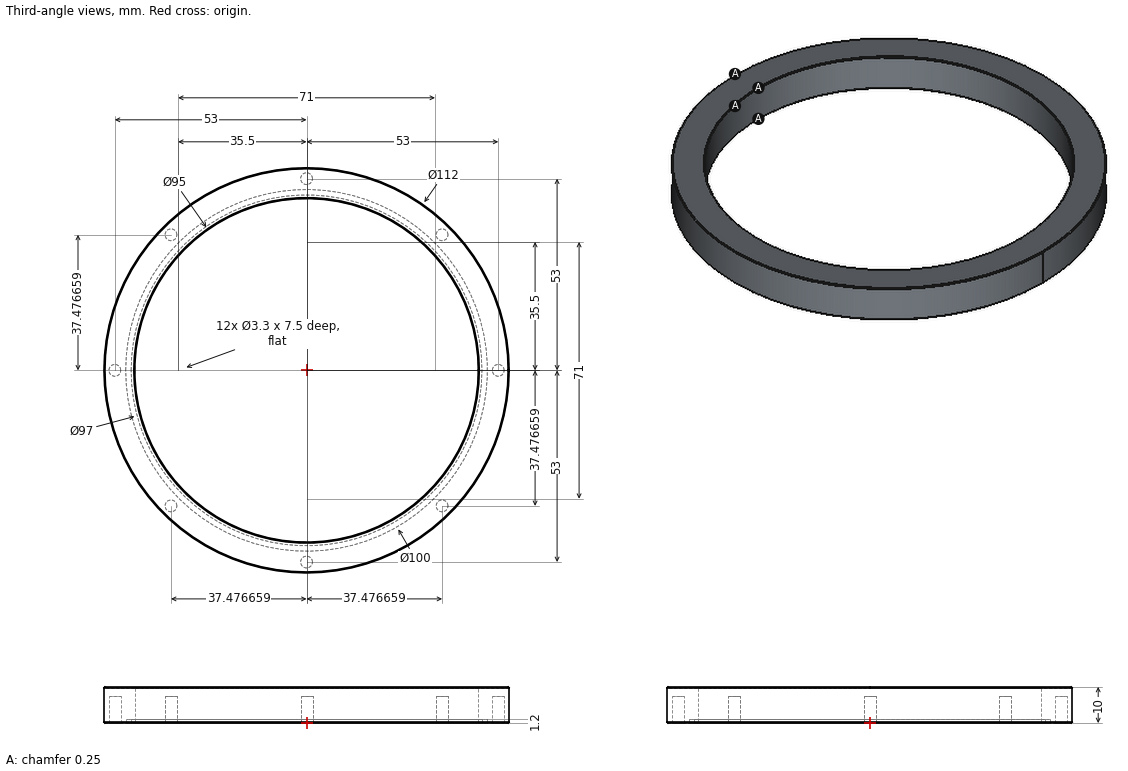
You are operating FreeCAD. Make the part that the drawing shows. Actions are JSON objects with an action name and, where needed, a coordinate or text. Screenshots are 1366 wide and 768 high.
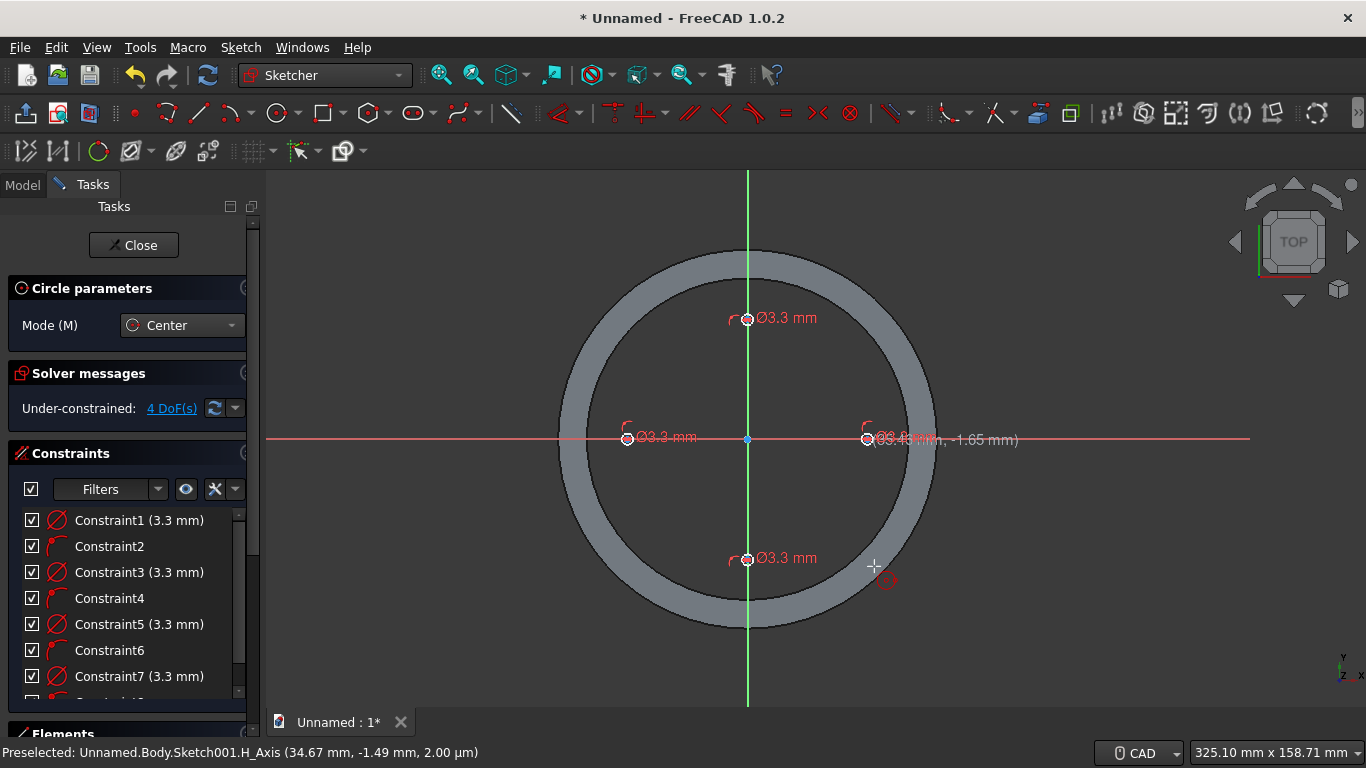
{"action": "left_click", "coordinate": [874, 566]}
{"action": "mouse_move", "coordinate": [878, 562]}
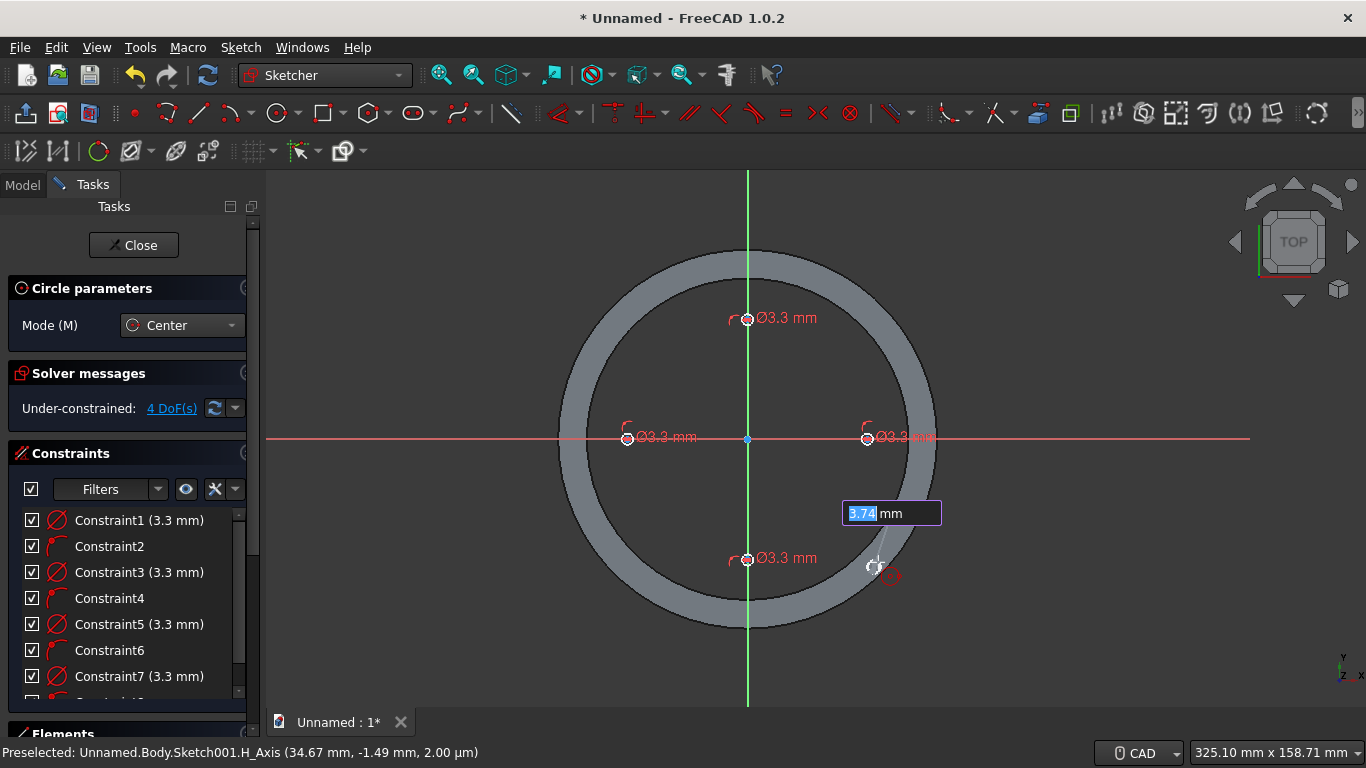
{"action": "type", "text": "3.3"}
{"action": "key", "text": "Return"}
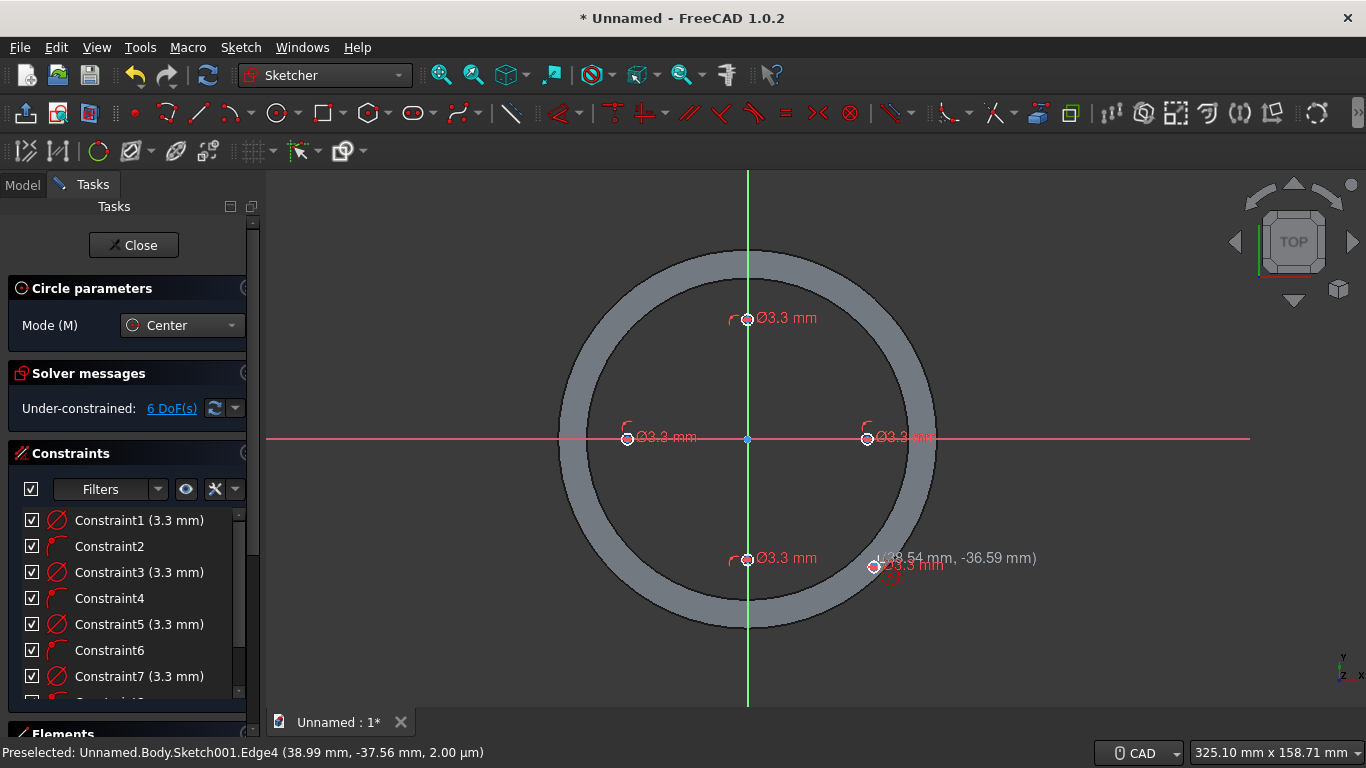
{"action": "scroll", "coordinate": [621, 566], "scroll_direction": "up", "scroll_amount": 8}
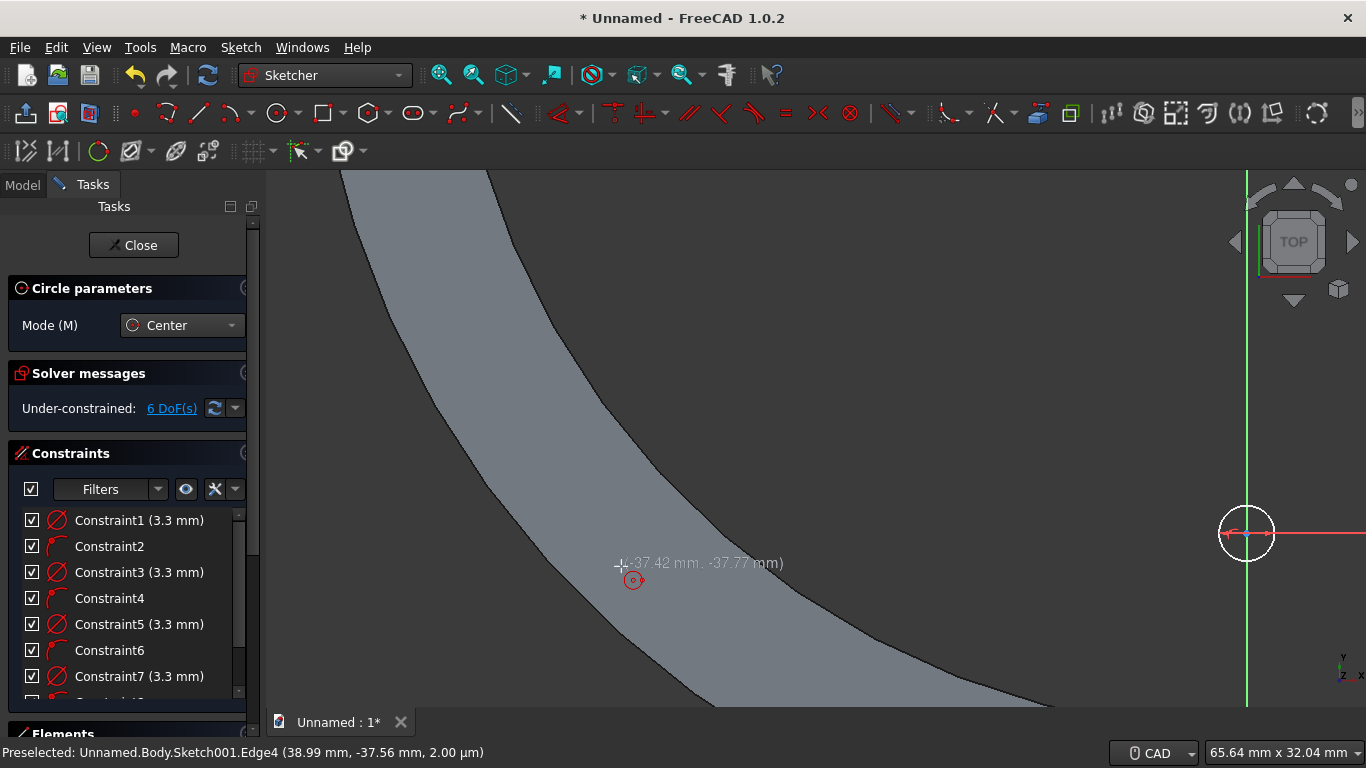
{"action": "scroll", "coordinate": [621, 566], "scroll_direction": "down", "scroll_amount": 8}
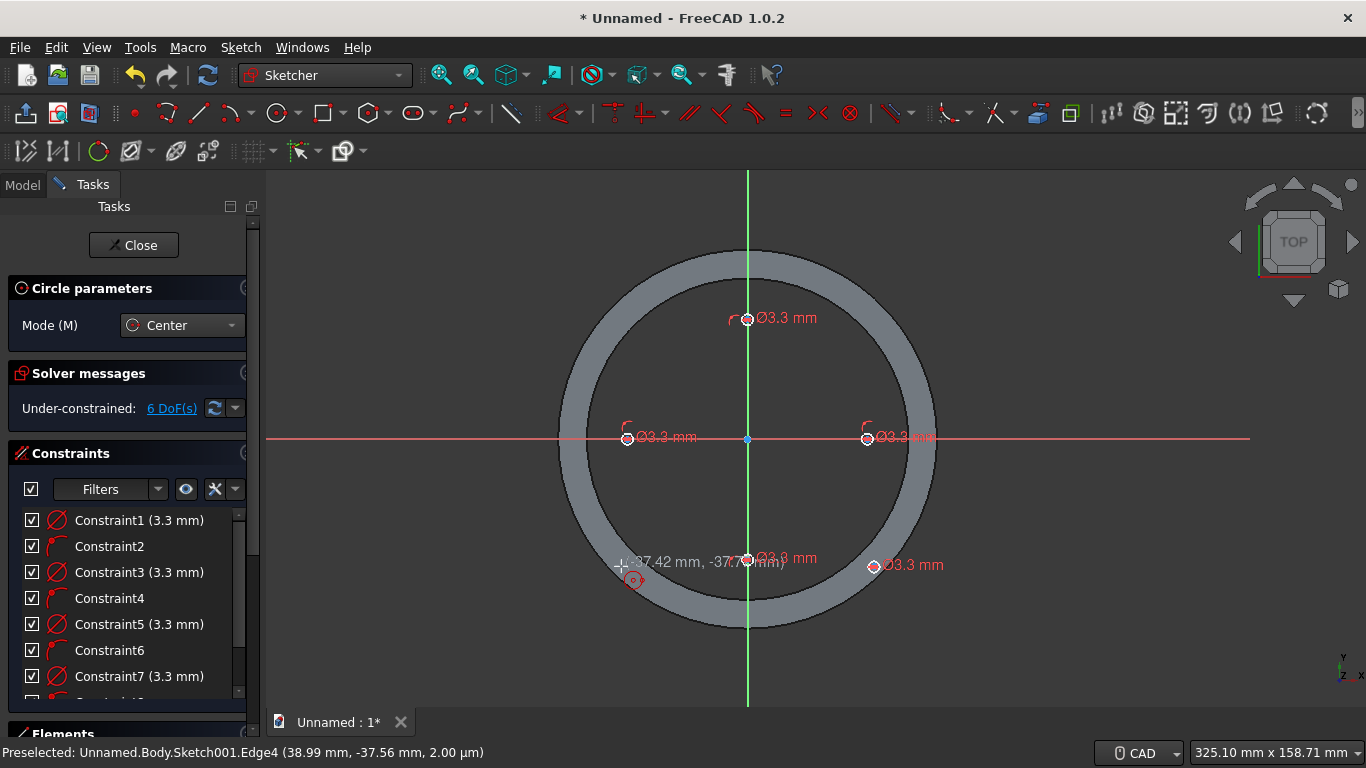
{"action": "left_click", "coordinate": [621, 566]}
{"action": "mouse_move", "coordinate": [625, 562]}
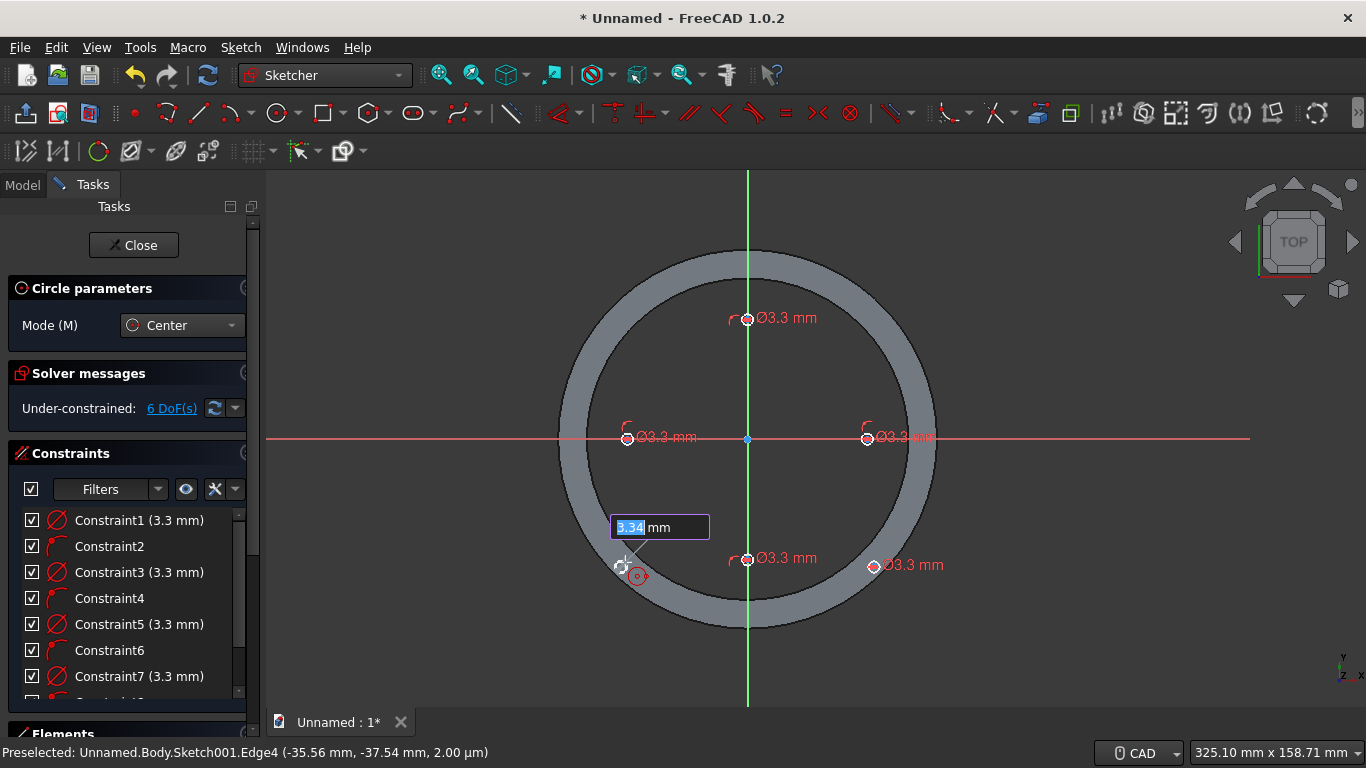
{"action": "type", "text": "3.3"}
{"action": "key", "text": "Return"}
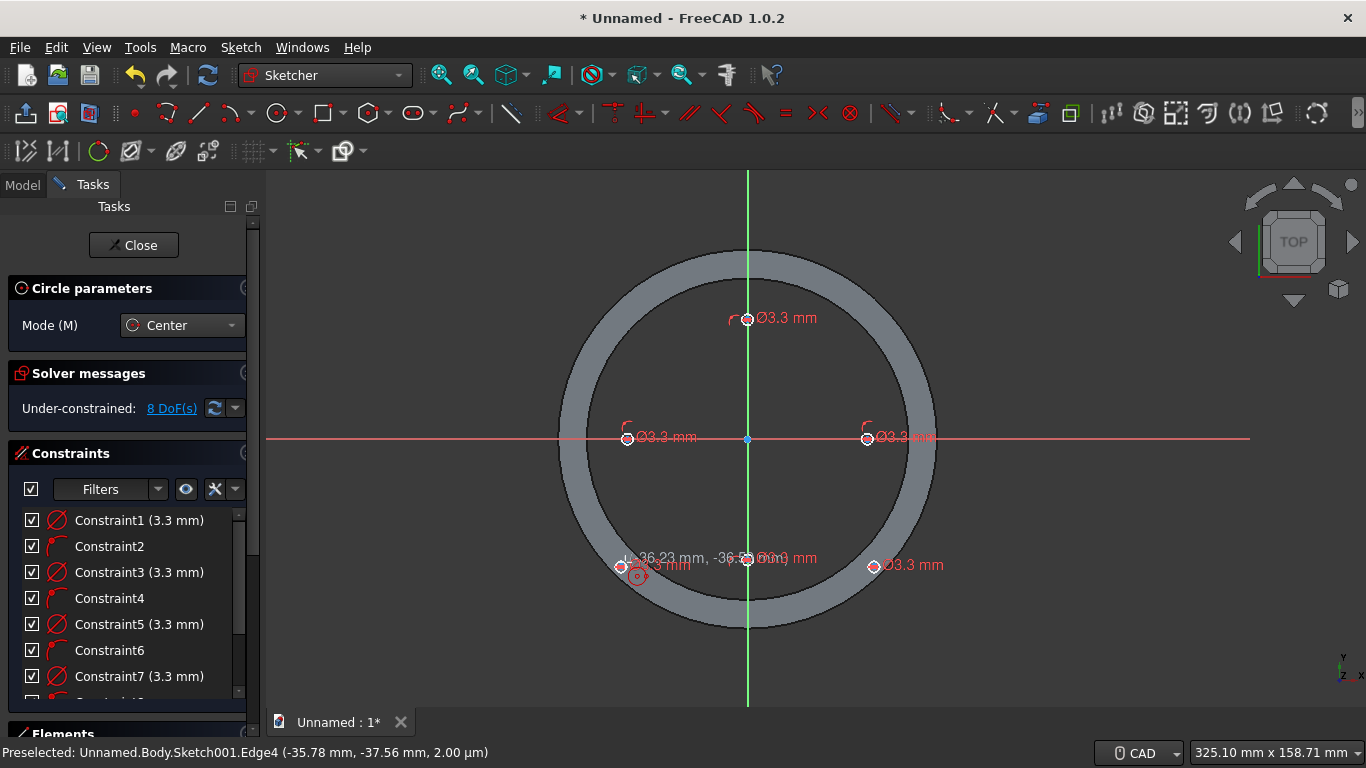
{"action": "scroll", "coordinate": [621, 312], "scroll_direction": "up", "scroll_amount": 8}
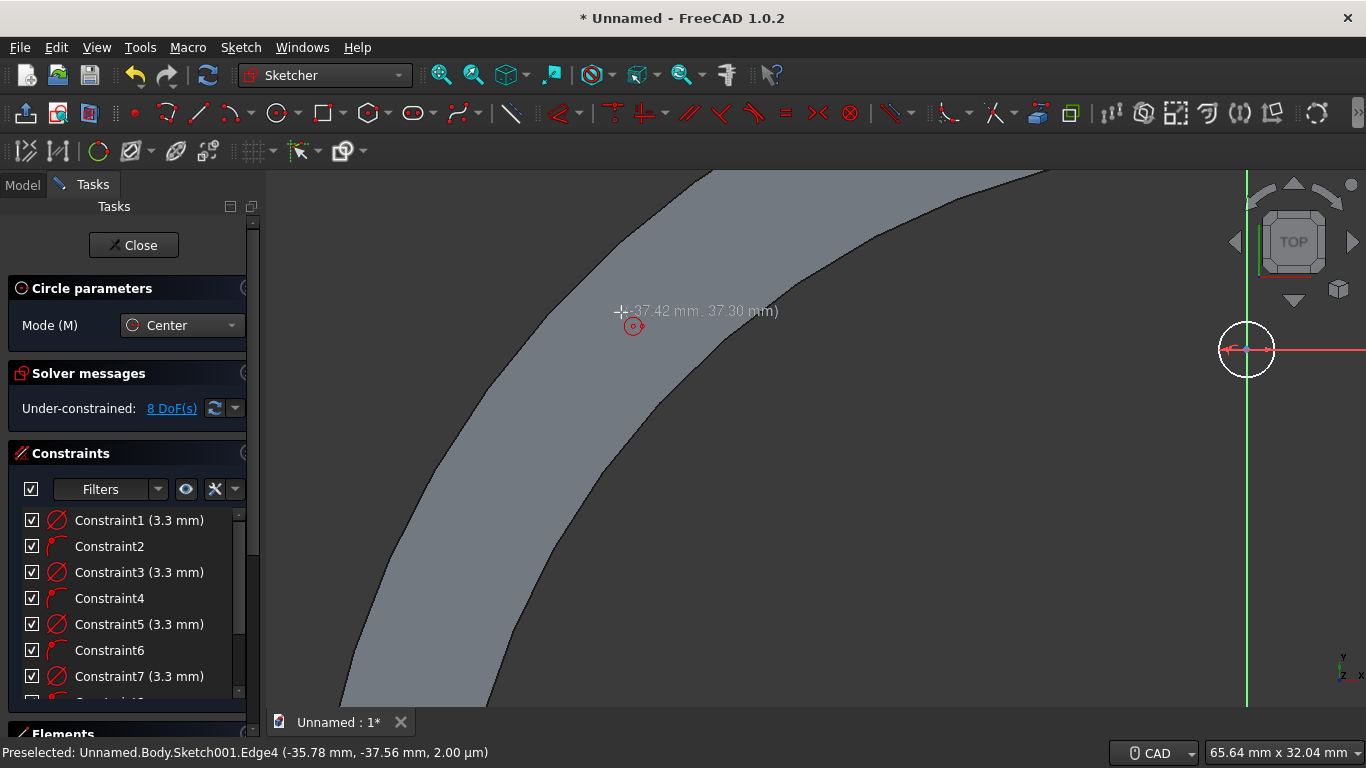
{"action": "scroll", "coordinate": [621, 311], "scroll_direction": "down", "scroll_amount": 8}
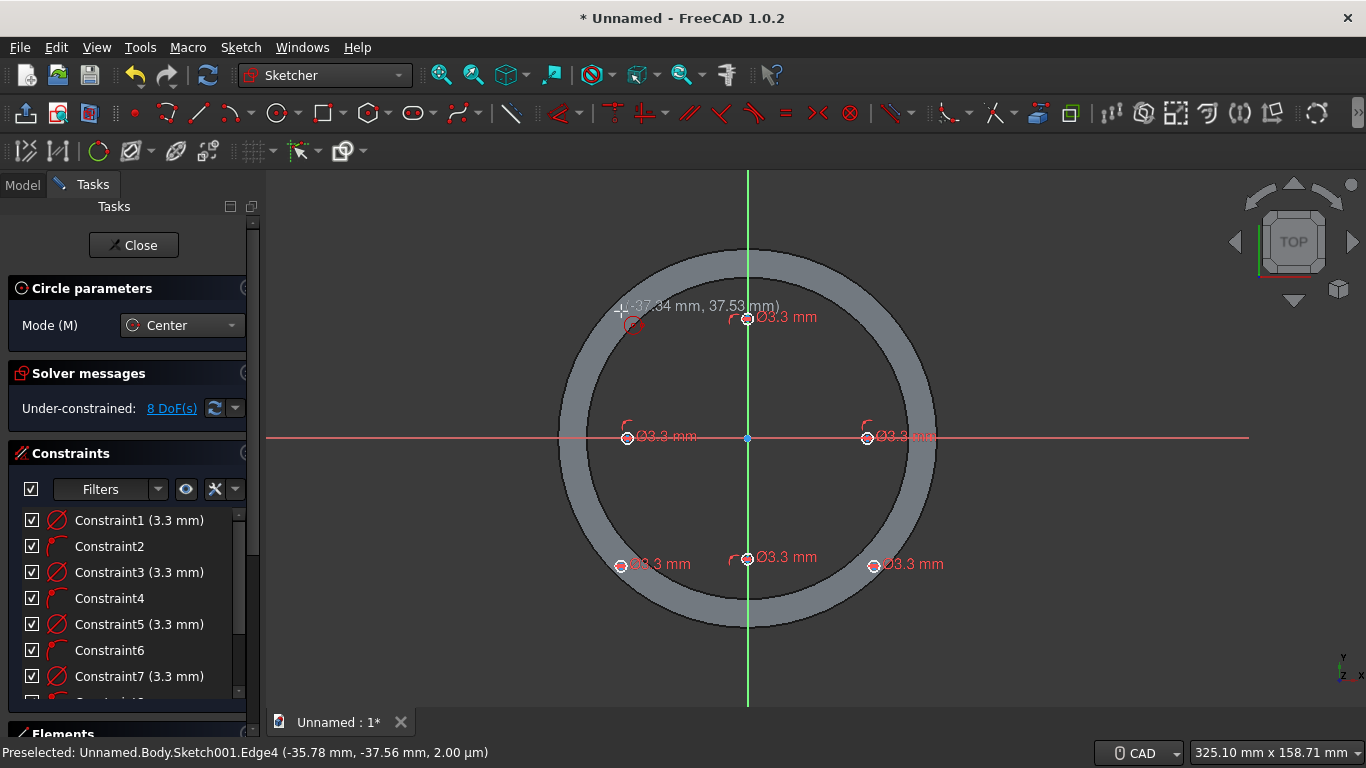
{"action": "left_click", "coordinate": [621, 312]}
{"action": "mouse_move", "coordinate": [625, 308]}